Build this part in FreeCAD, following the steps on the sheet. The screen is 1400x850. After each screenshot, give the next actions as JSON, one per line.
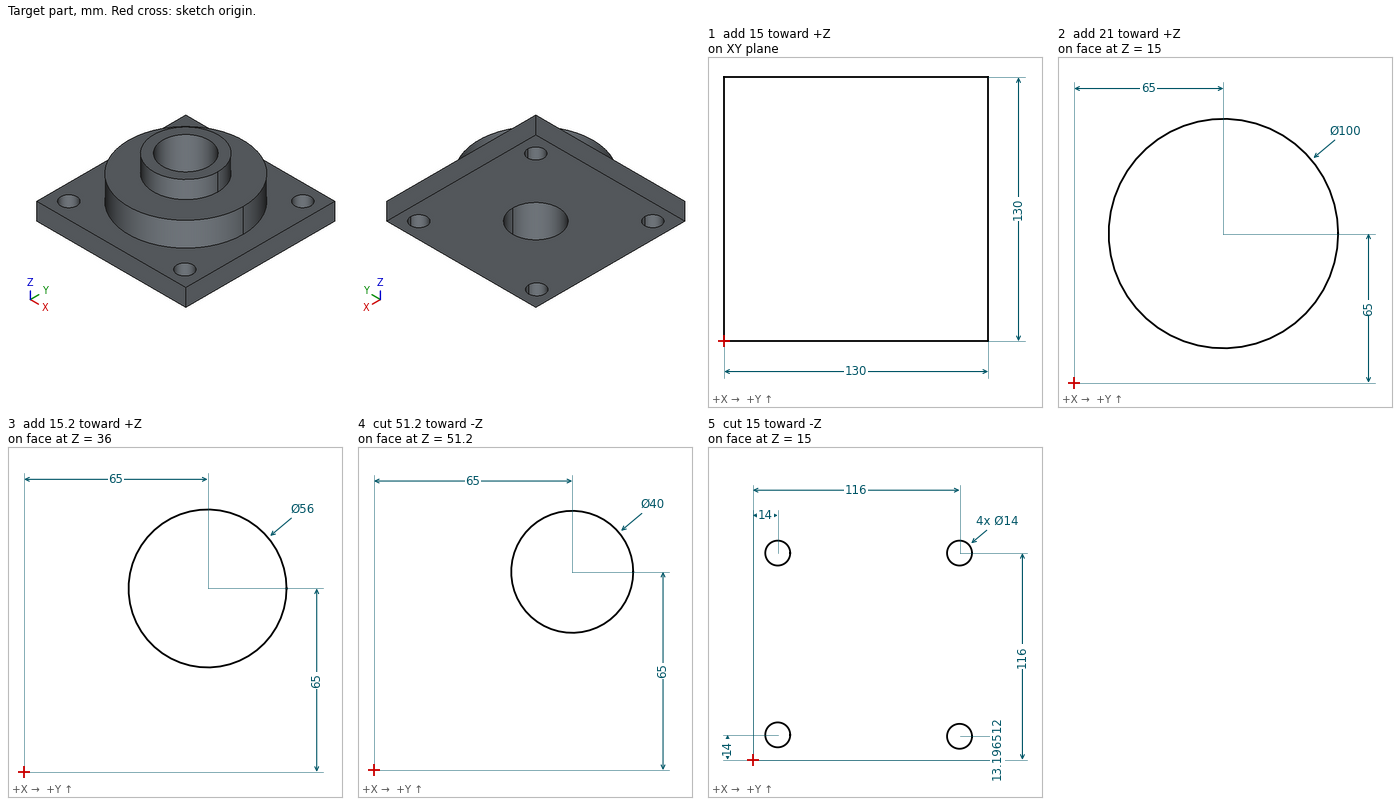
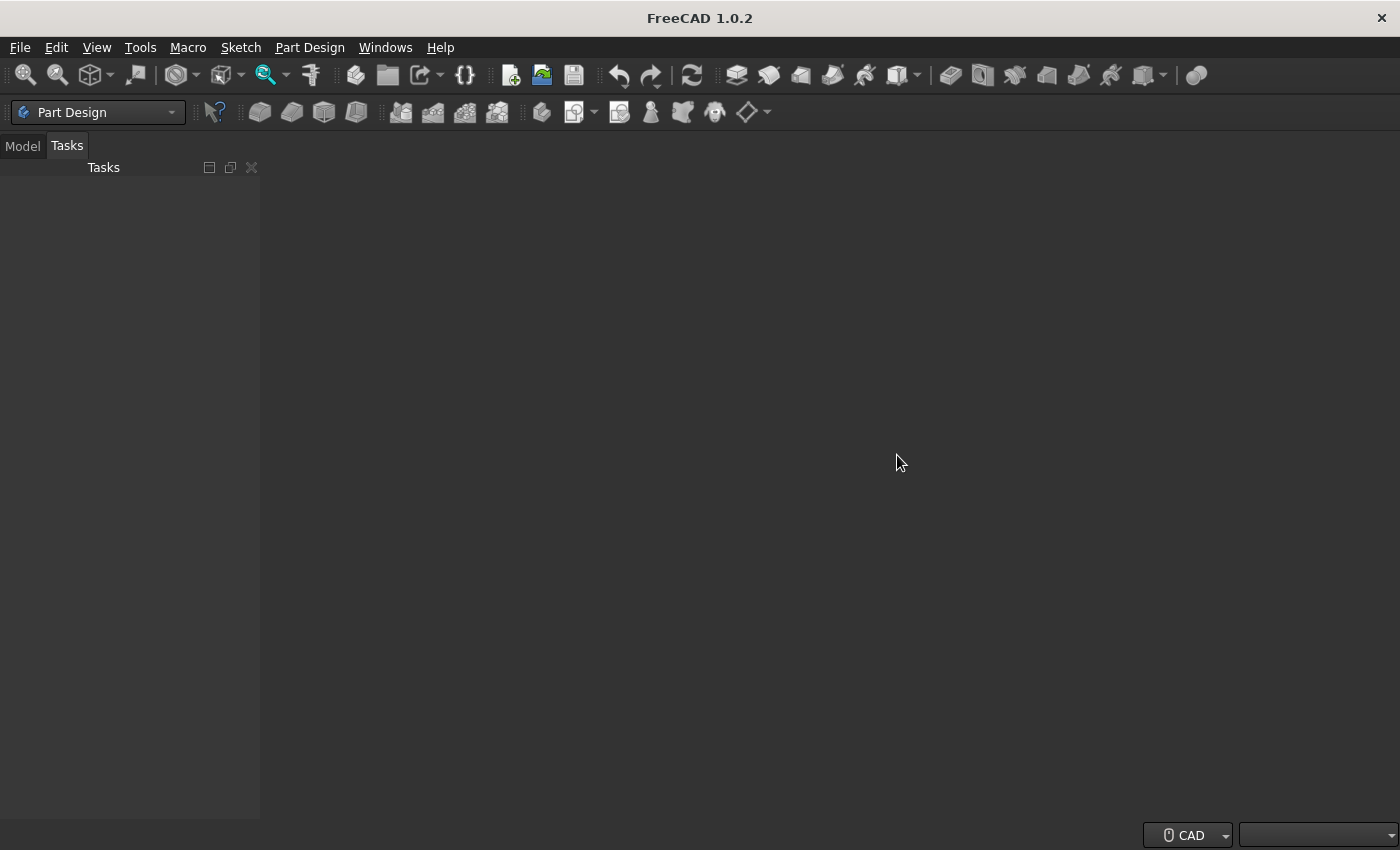
{"action": "left_click", "coordinate": [510, 76]}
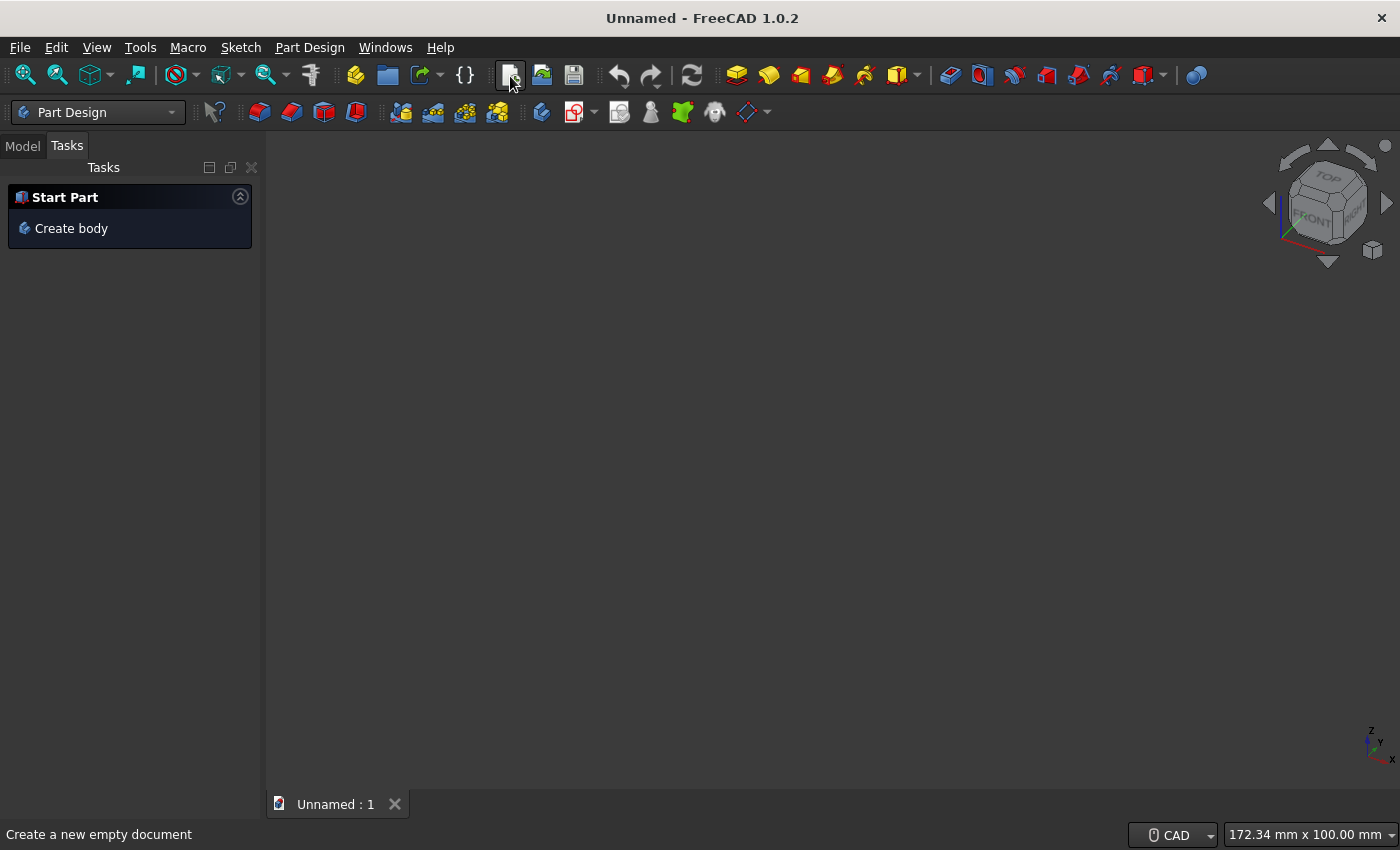
{"action": "left_click", "coordinate": [574, 112]}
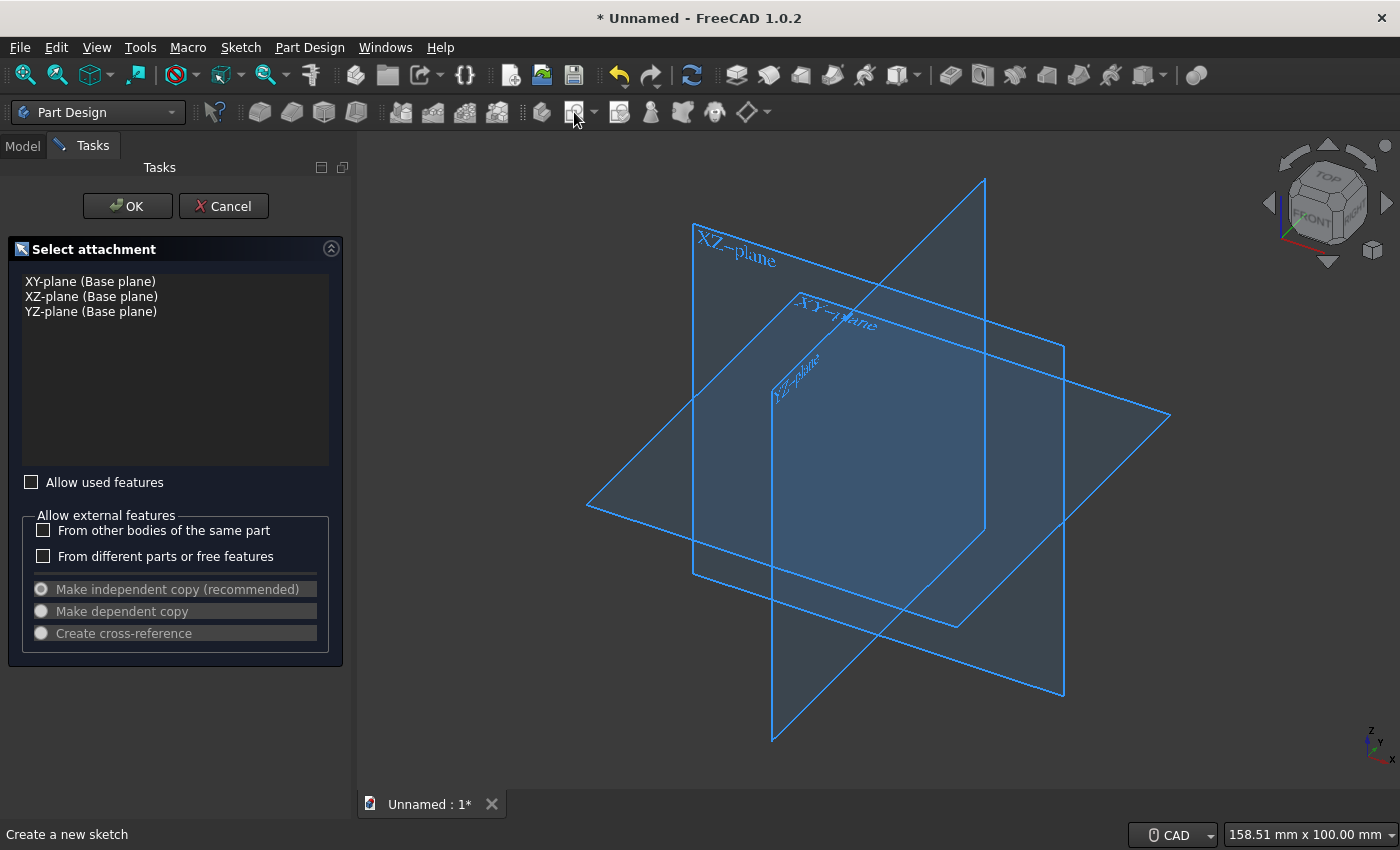
{"action": "left_click", "coordinate": [82, 282]}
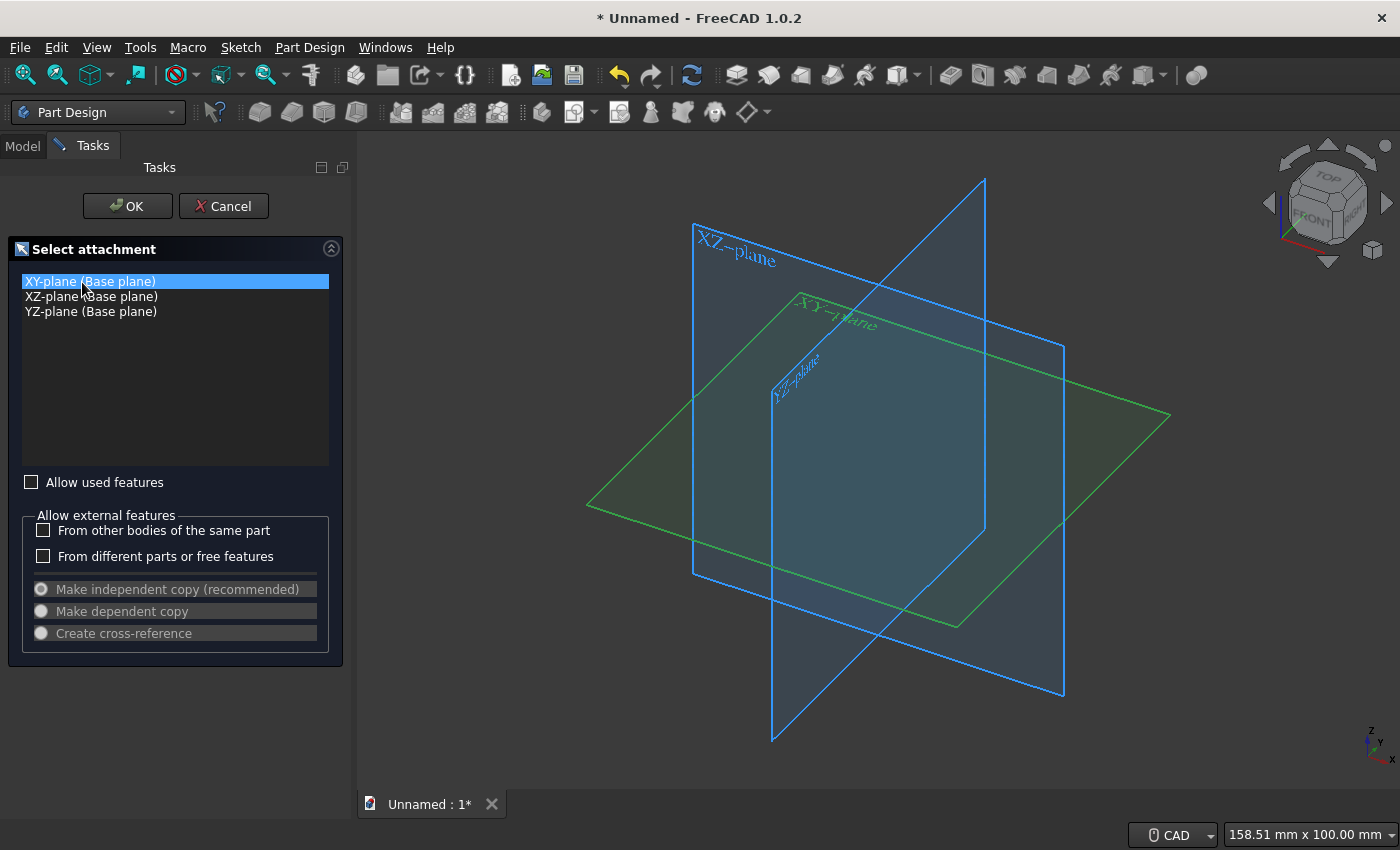
{"action": "left_click", "coordinate": [128, 206]}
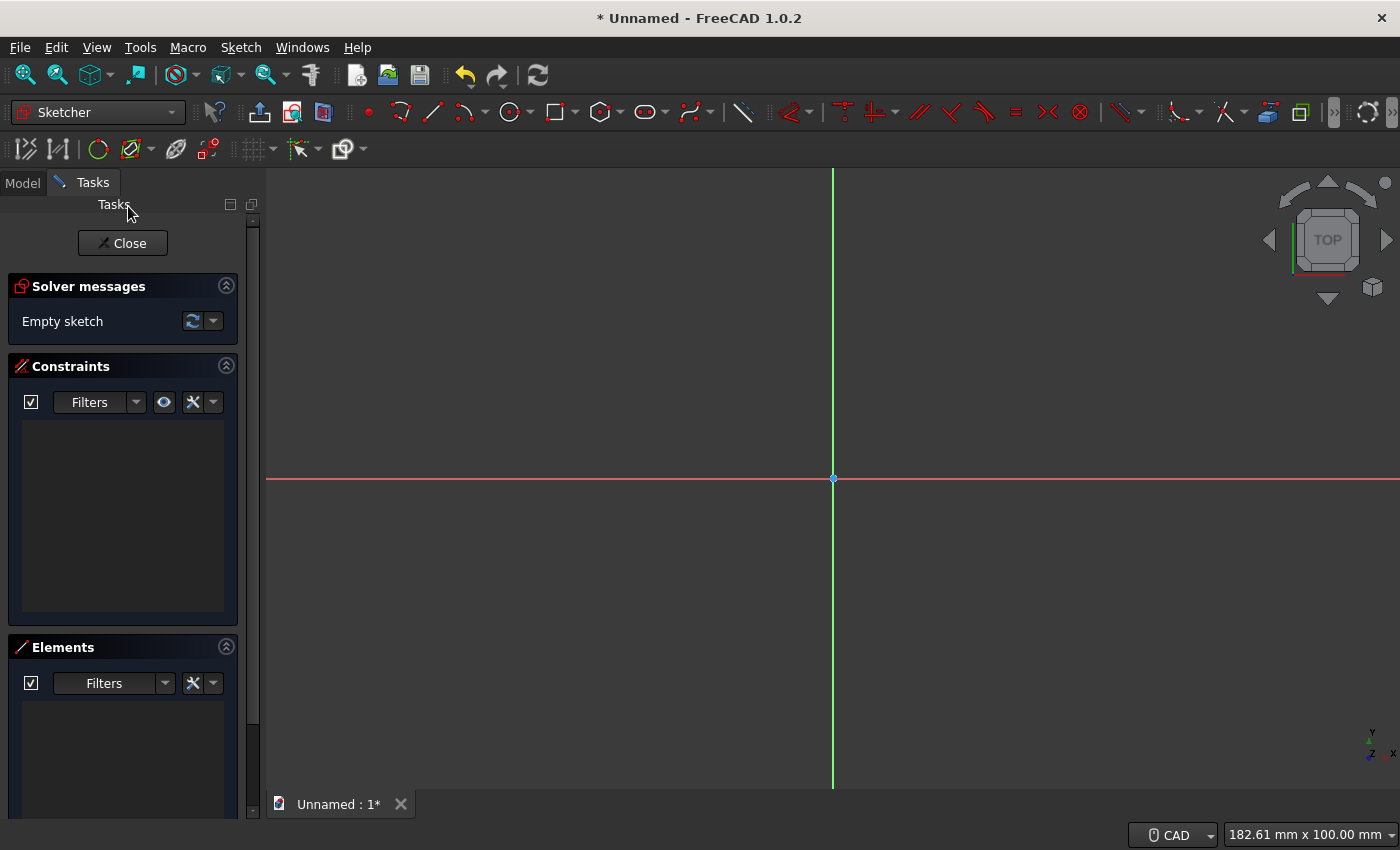
{"action": "scroll", "coordinate": [379, 761], "scroll_direction": "down", "scroll_amount": 4}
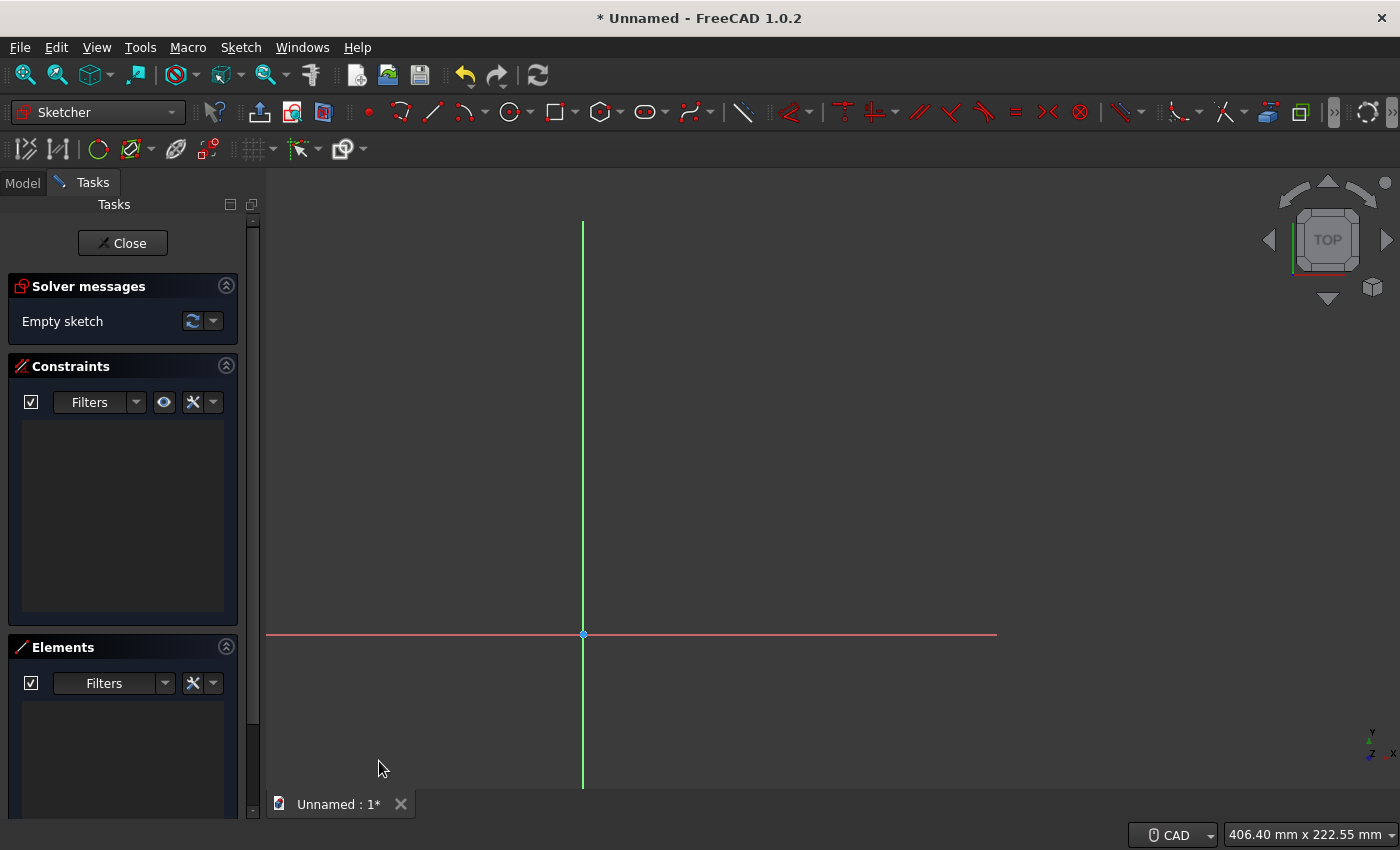
{"action": "key", "text": "g r"}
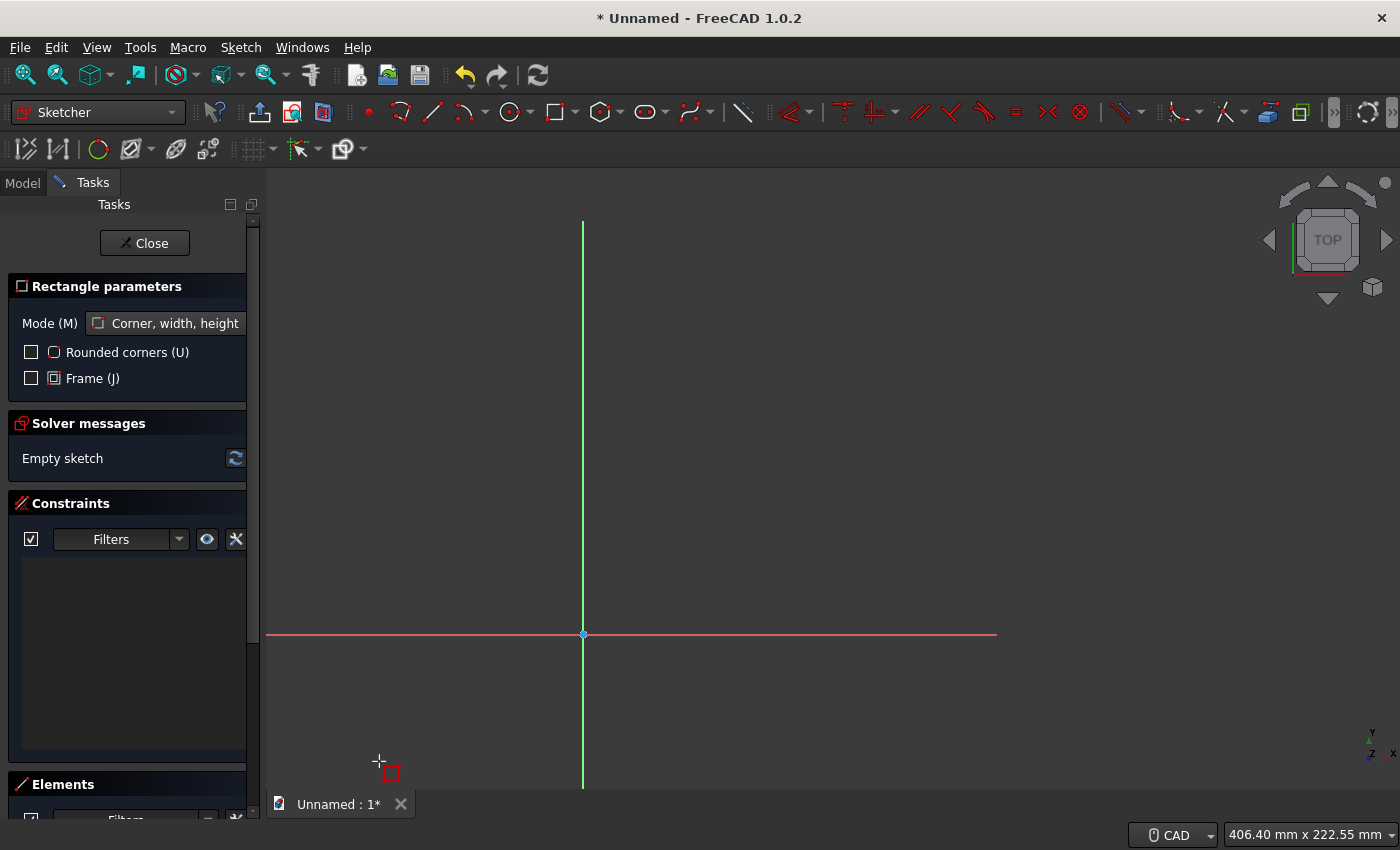
{"action": "left_click", "coordinate": [583, 635]}
{"action": "mouse_move", "coordinate": [946, 272]}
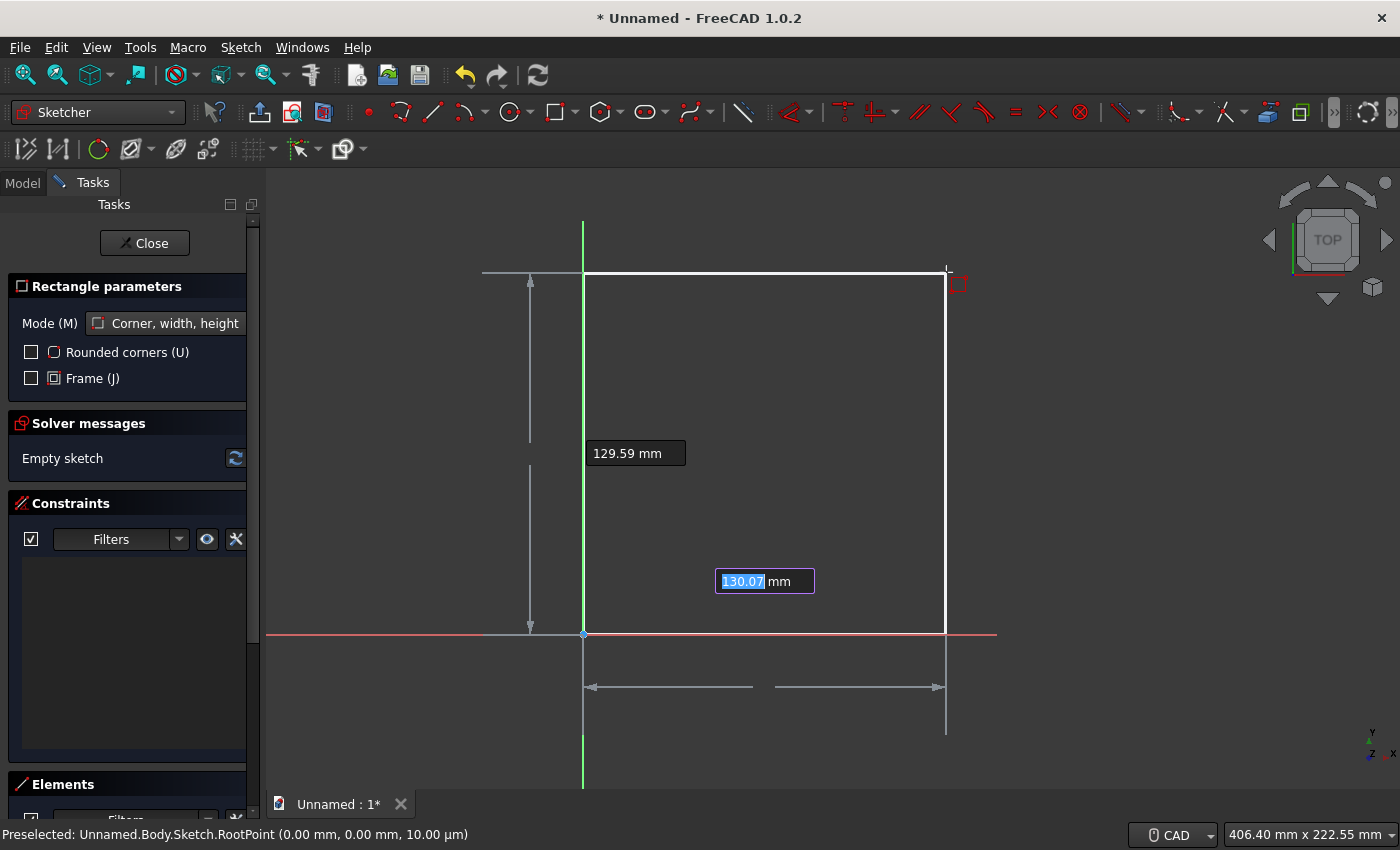
{"action": "type", "text": "130"}
{"action": "key", "text": "Tab"}
{"action": "type", "text": "130"}
{"action": "key", "text": "Return"}
{"action": "key", "text": "Escape"}